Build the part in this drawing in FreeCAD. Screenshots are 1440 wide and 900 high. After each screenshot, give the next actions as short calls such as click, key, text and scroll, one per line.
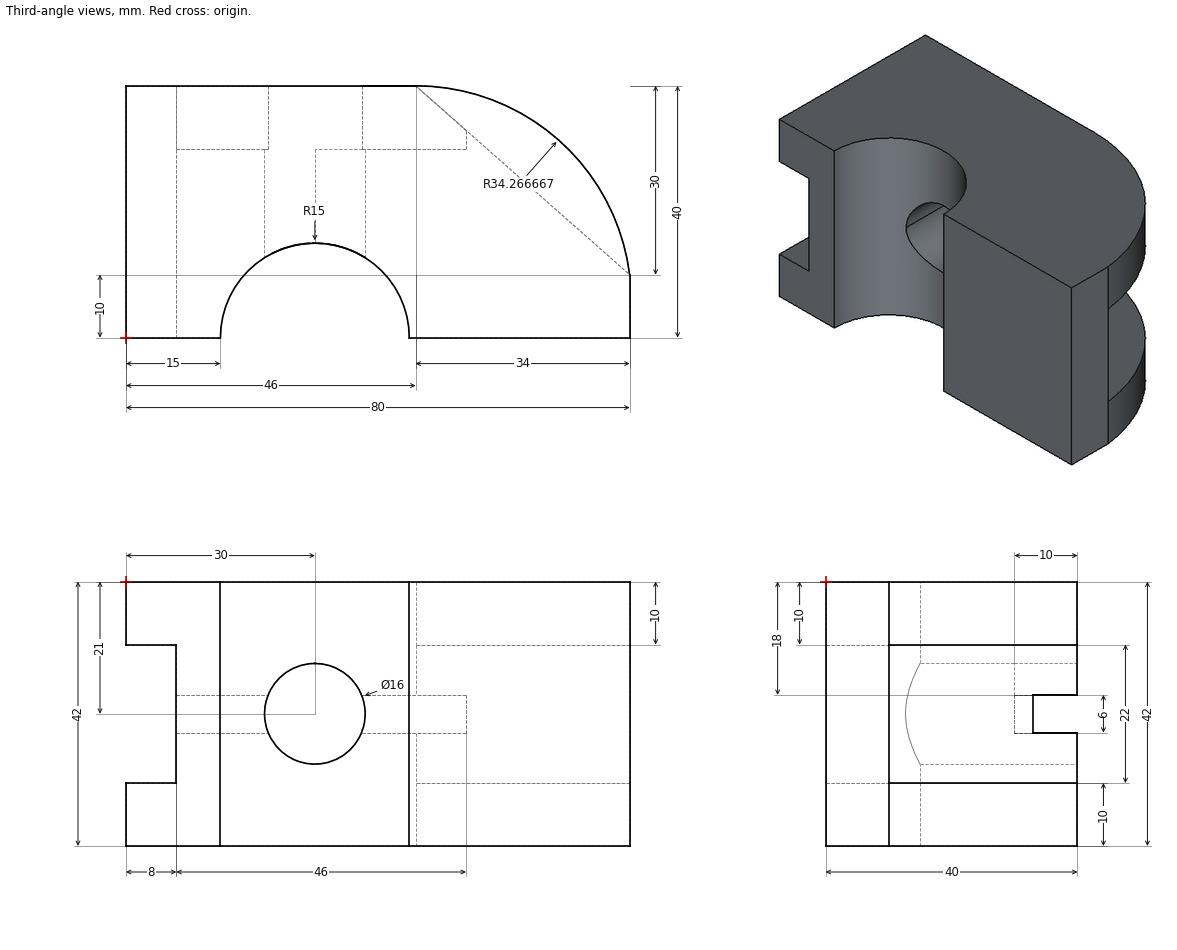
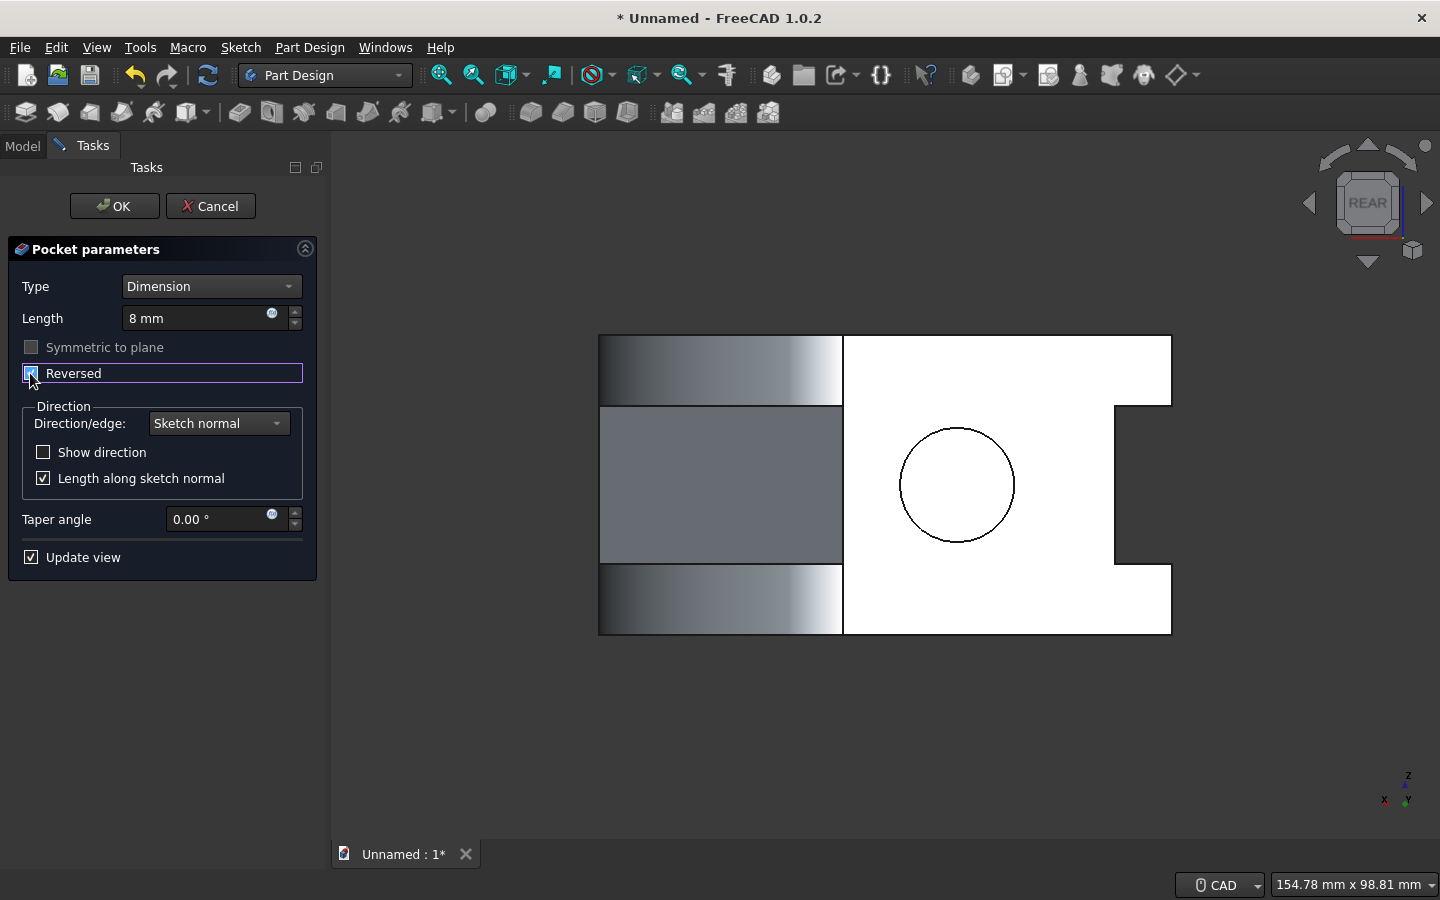
click(115, 206)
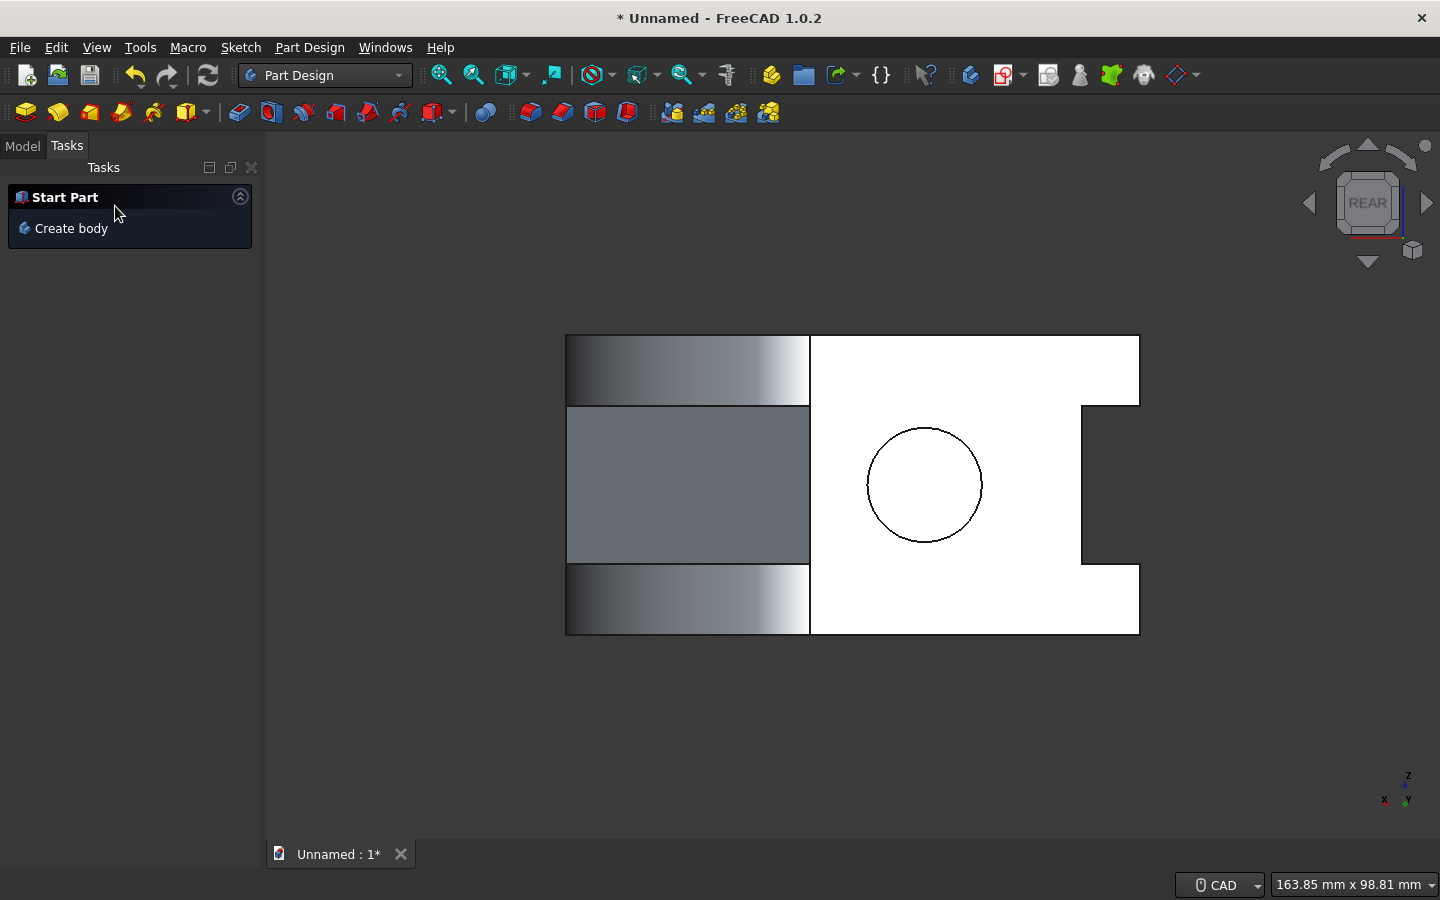
key(6)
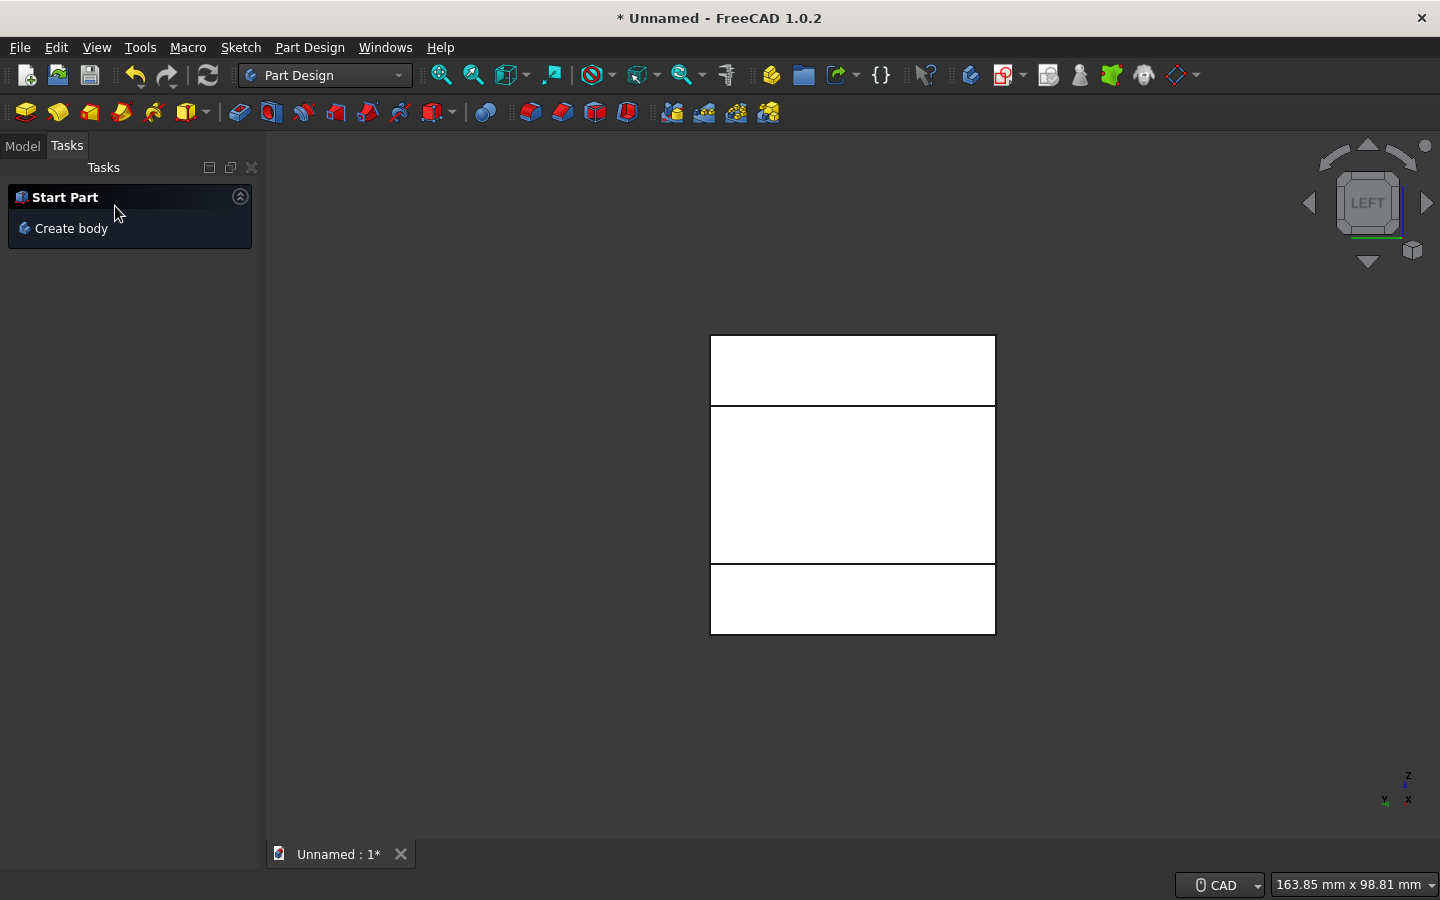
click(442, 76)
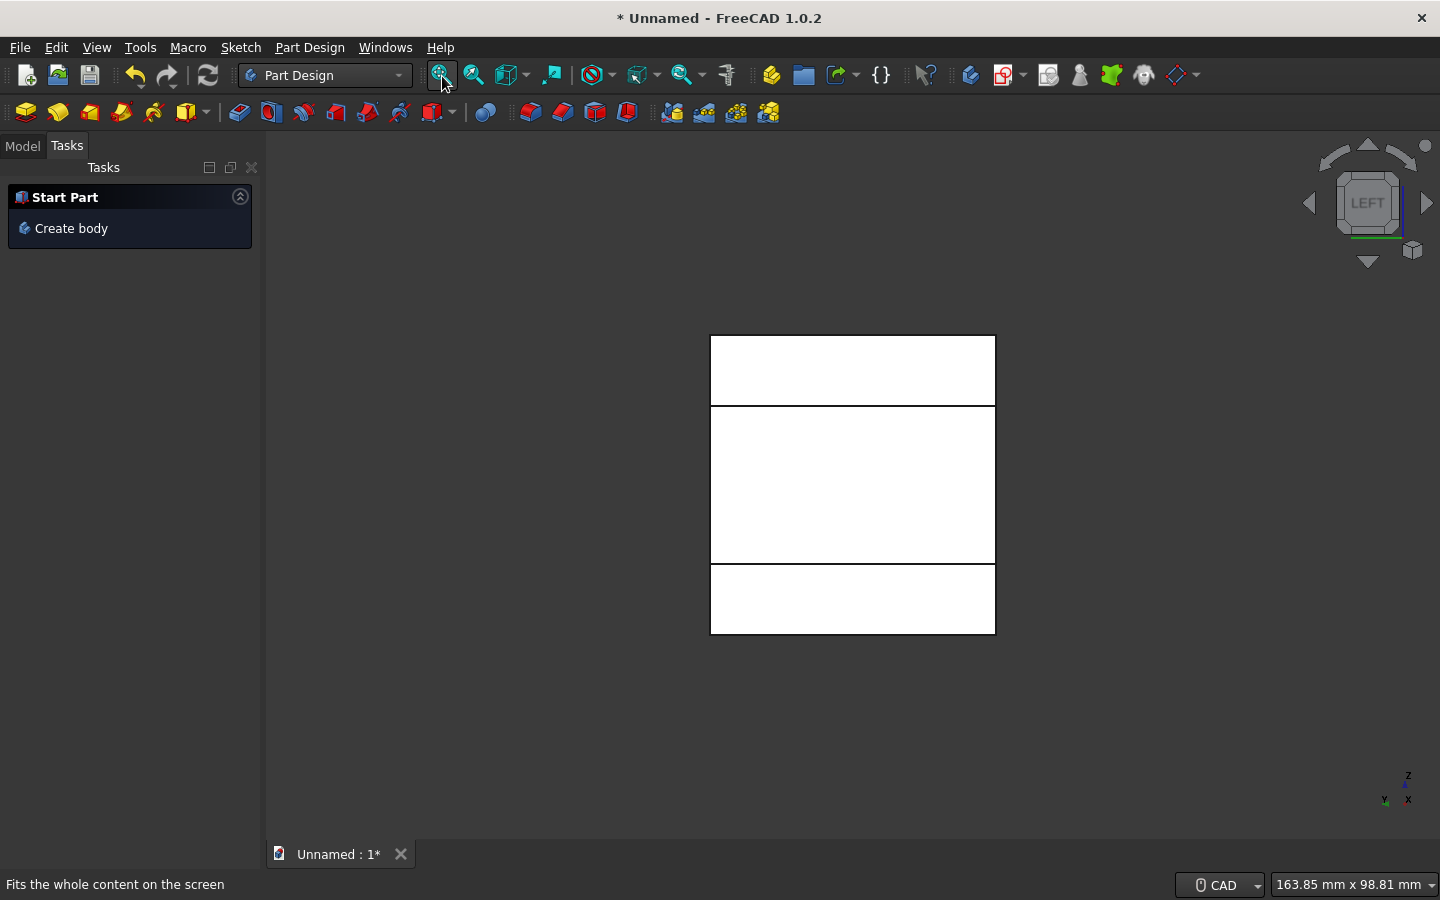
click(812, 484)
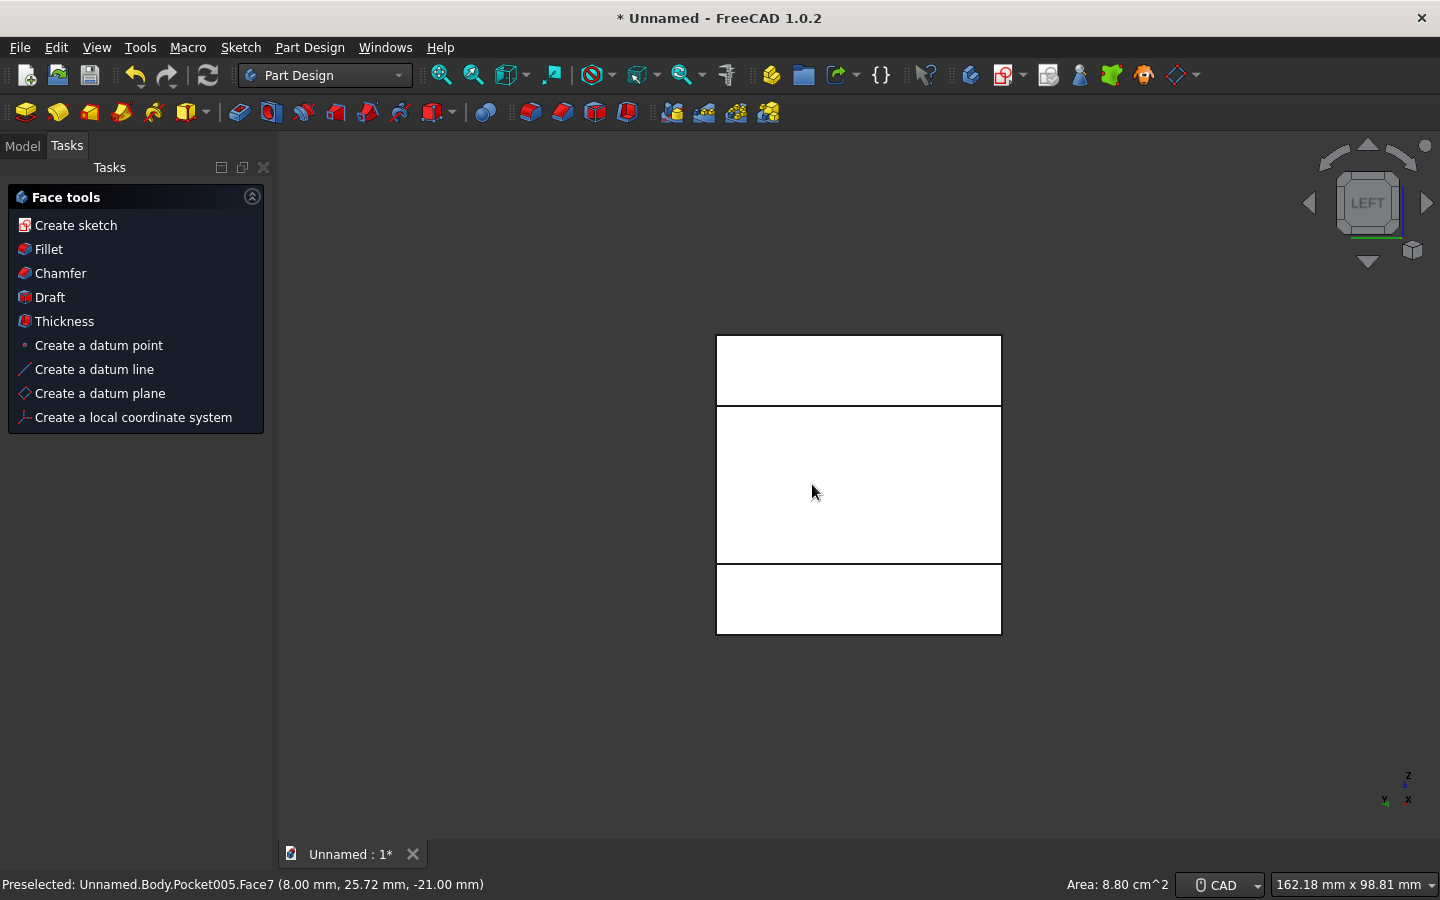
click(1004, 76)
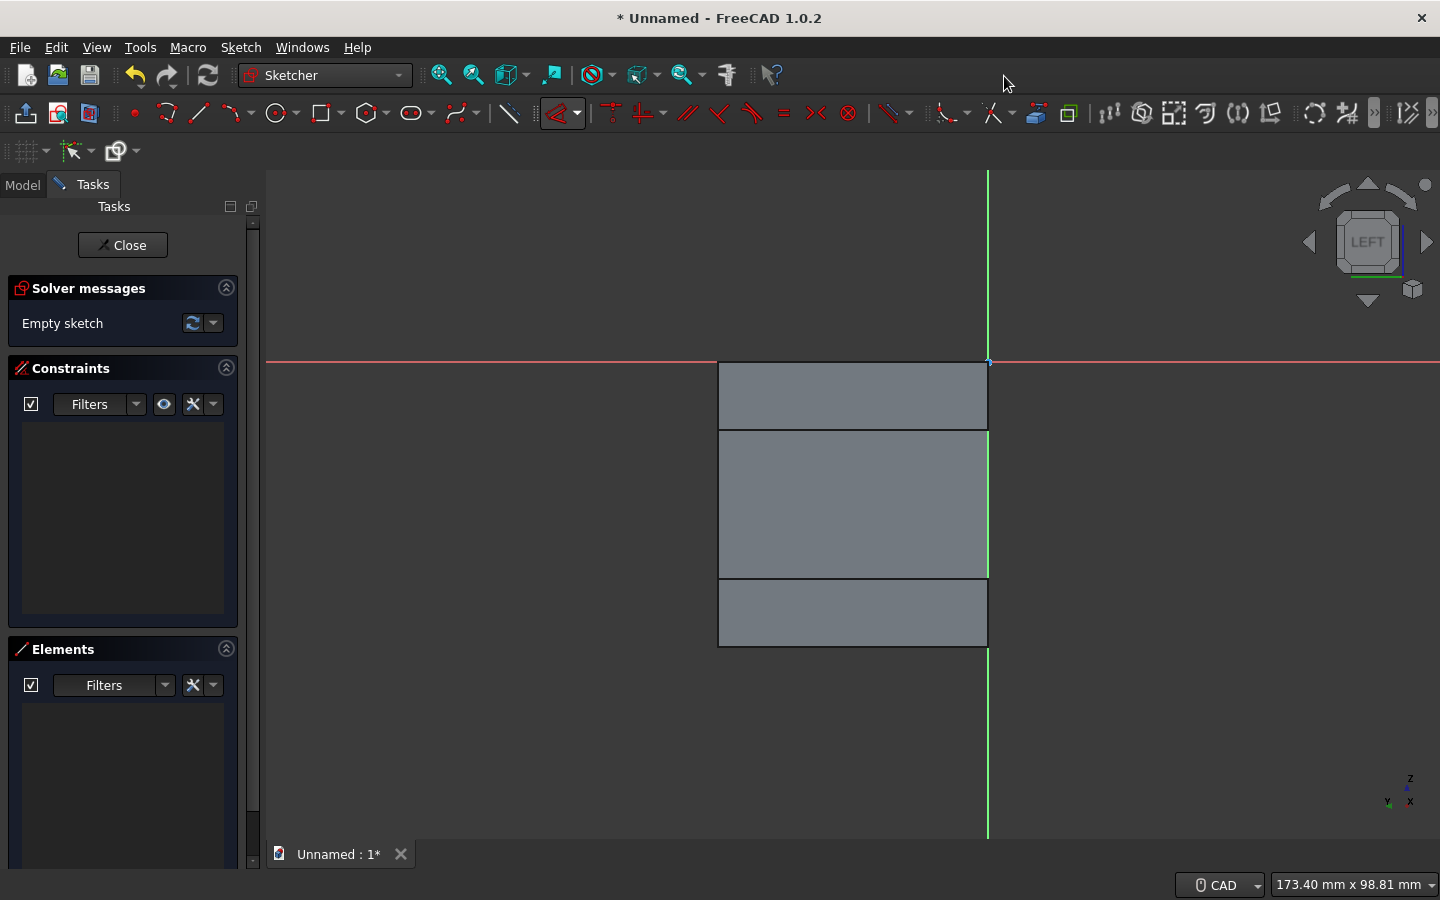
click(90, 114)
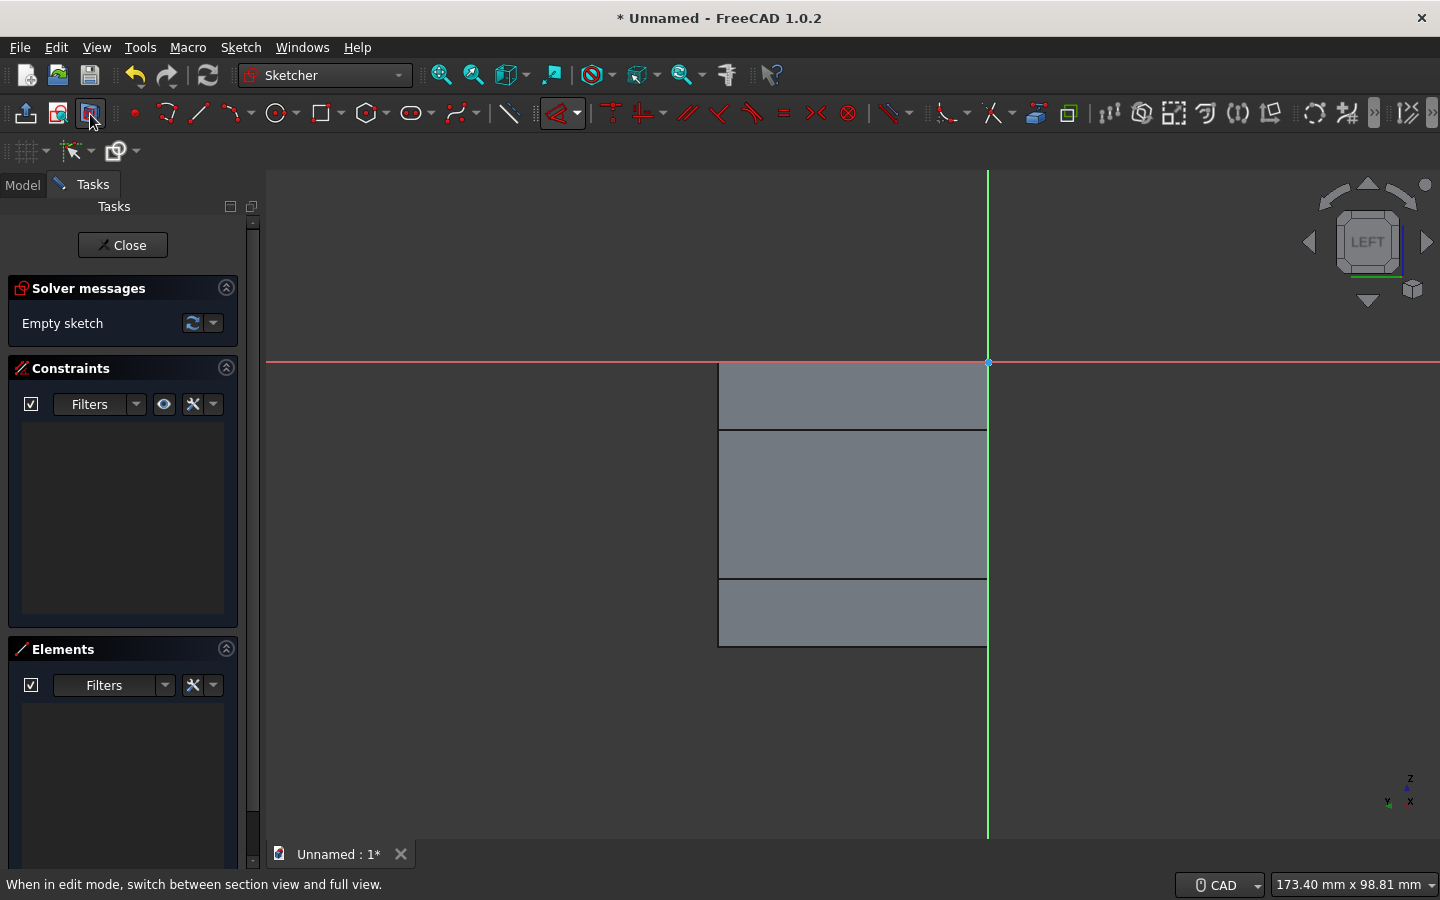
scroll(748, 504, up, 12)